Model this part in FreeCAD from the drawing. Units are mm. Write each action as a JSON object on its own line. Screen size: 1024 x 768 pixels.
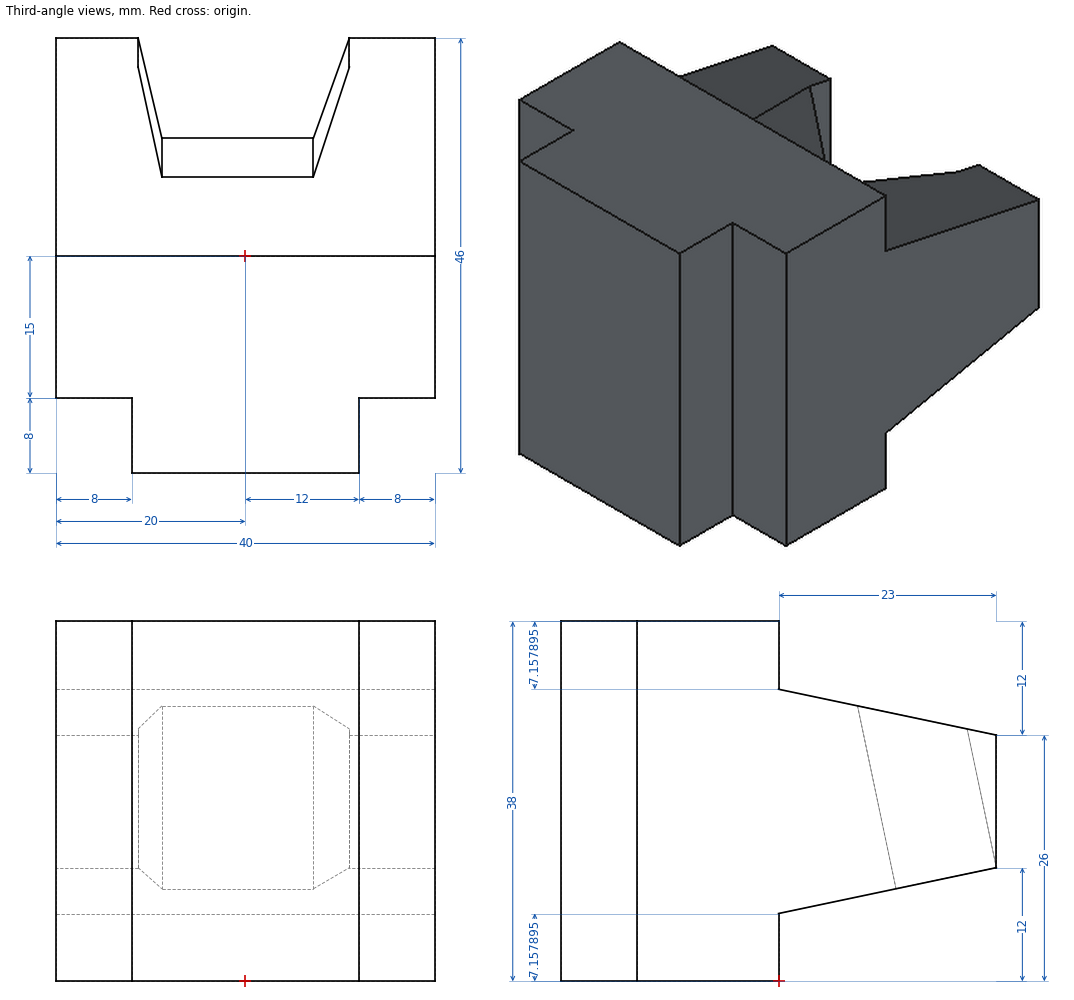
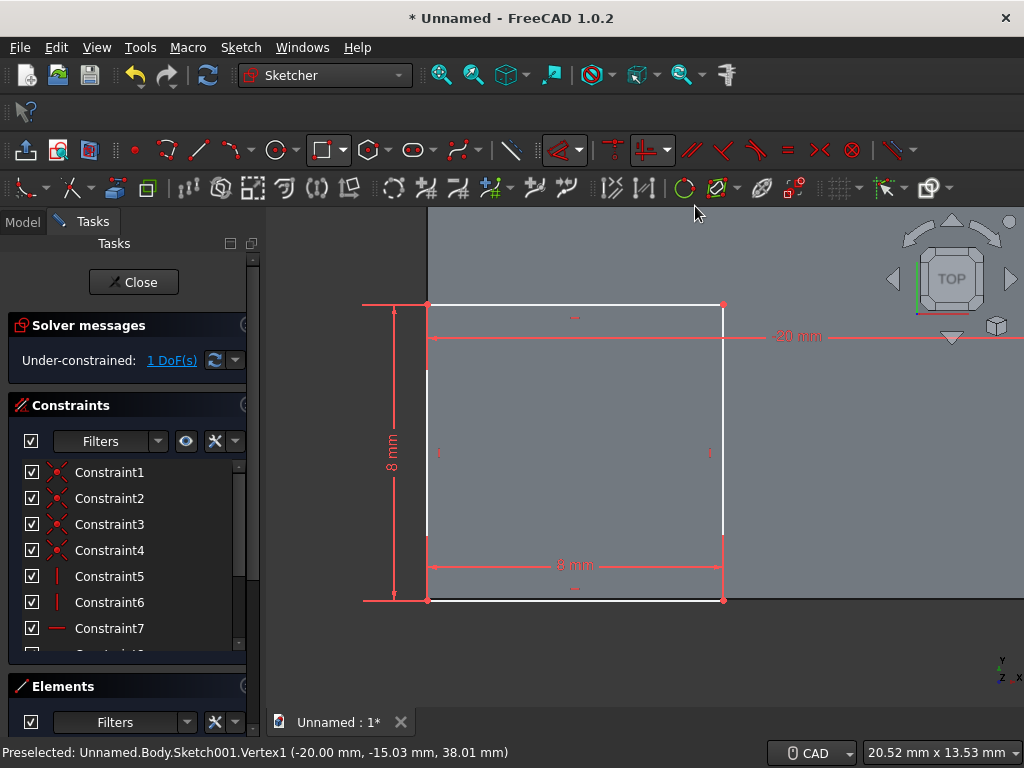
{"action": "left_click", "coordinate": [427, 305]}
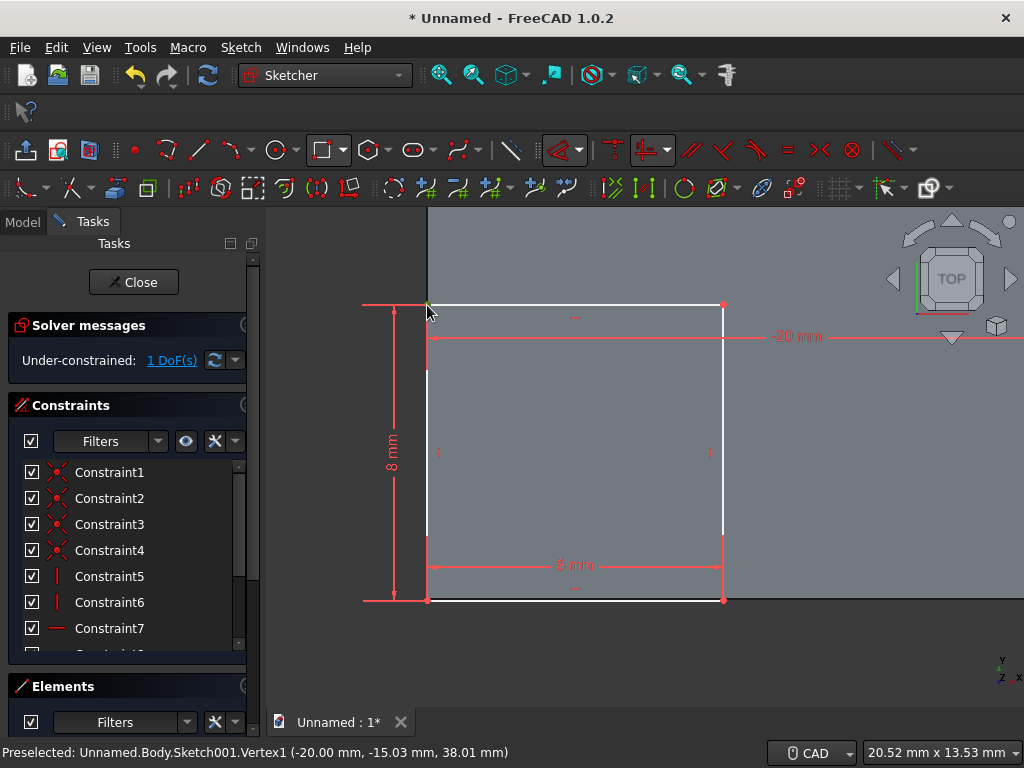
{"action": "left_click", "coordinate": [582, 150]}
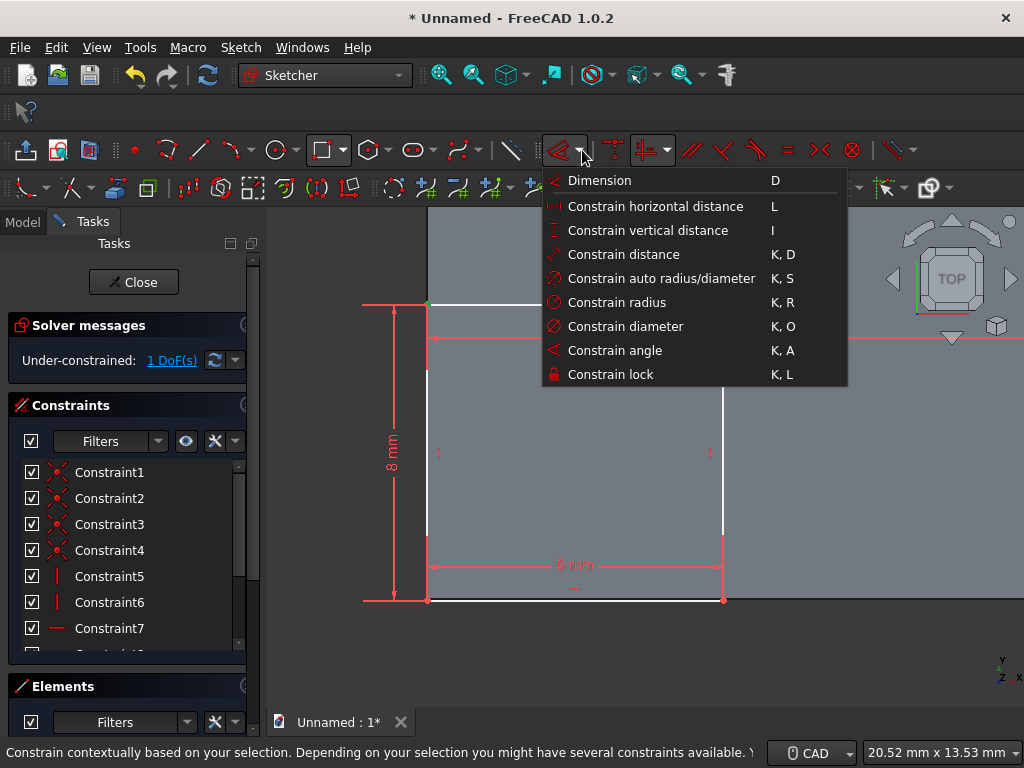
{"action": "left_click", "coordinate": [695, 230]}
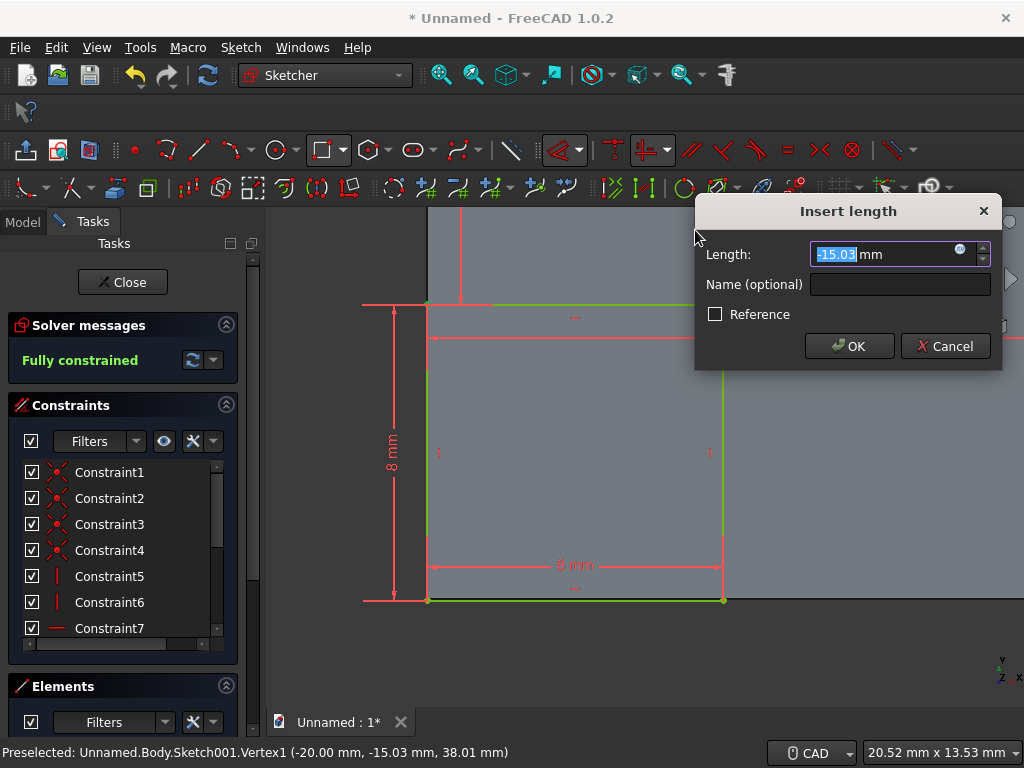
{"action": "type", "text": "-15"}
{"action": "key", "text": "Return"}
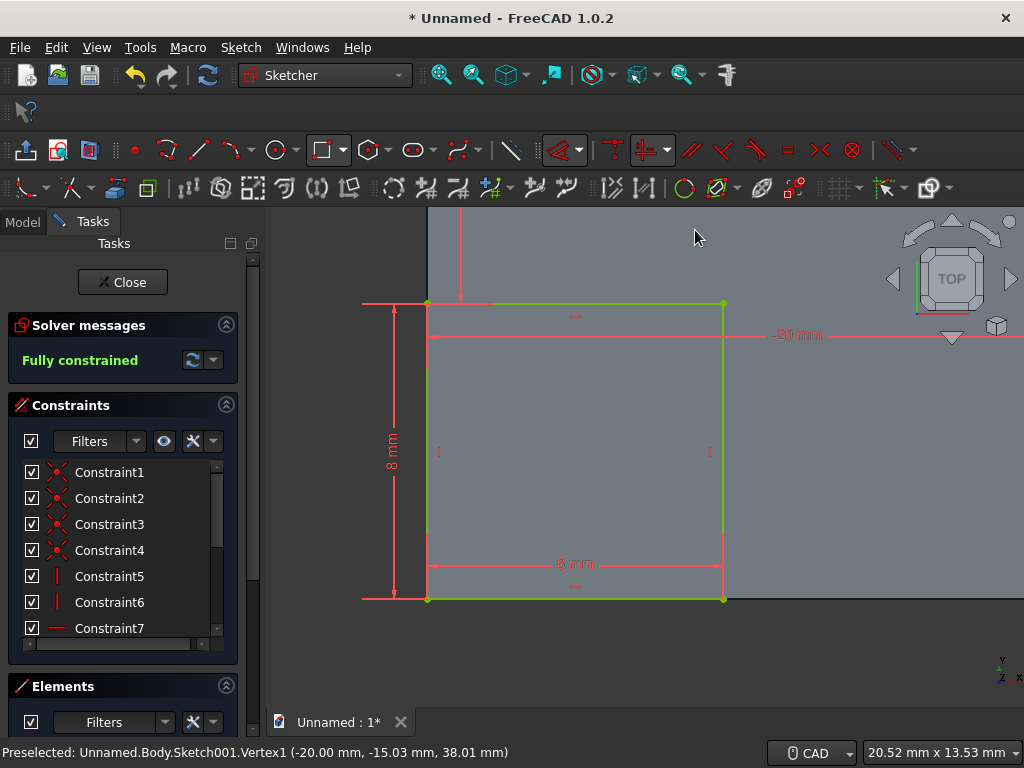
{"action": "left_click", "coordinate": [123, 282]}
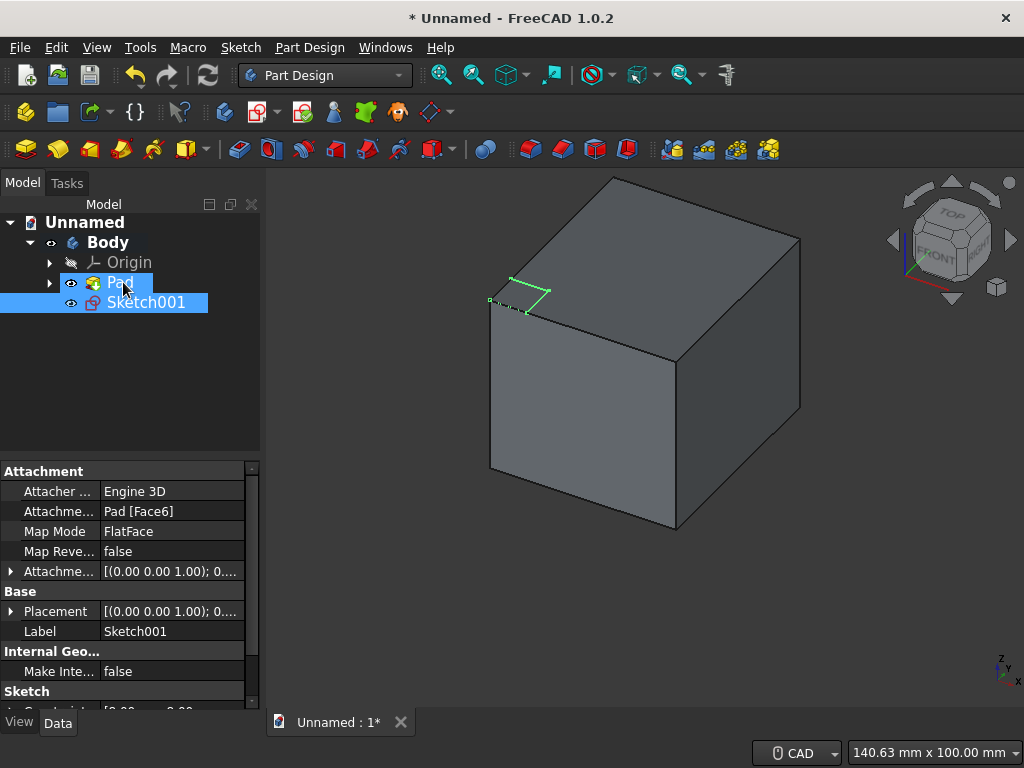
{"action": "left_click", "coordinate": [240, 150]}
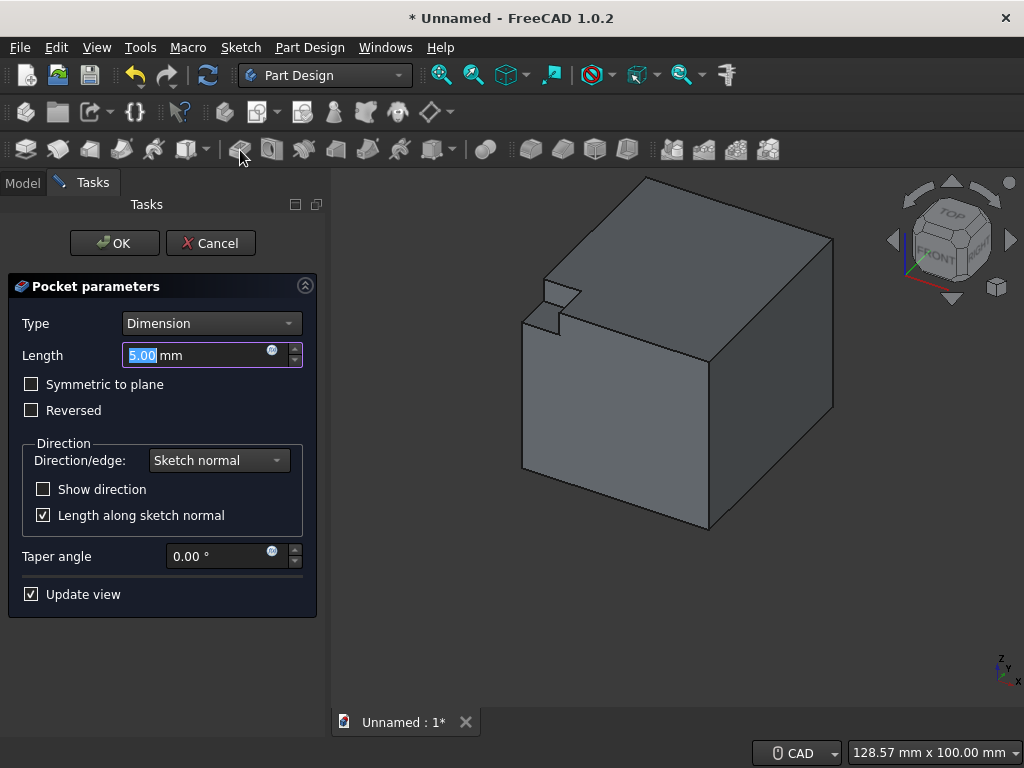
{"action": "left_click", "coordinate": [212, 324]}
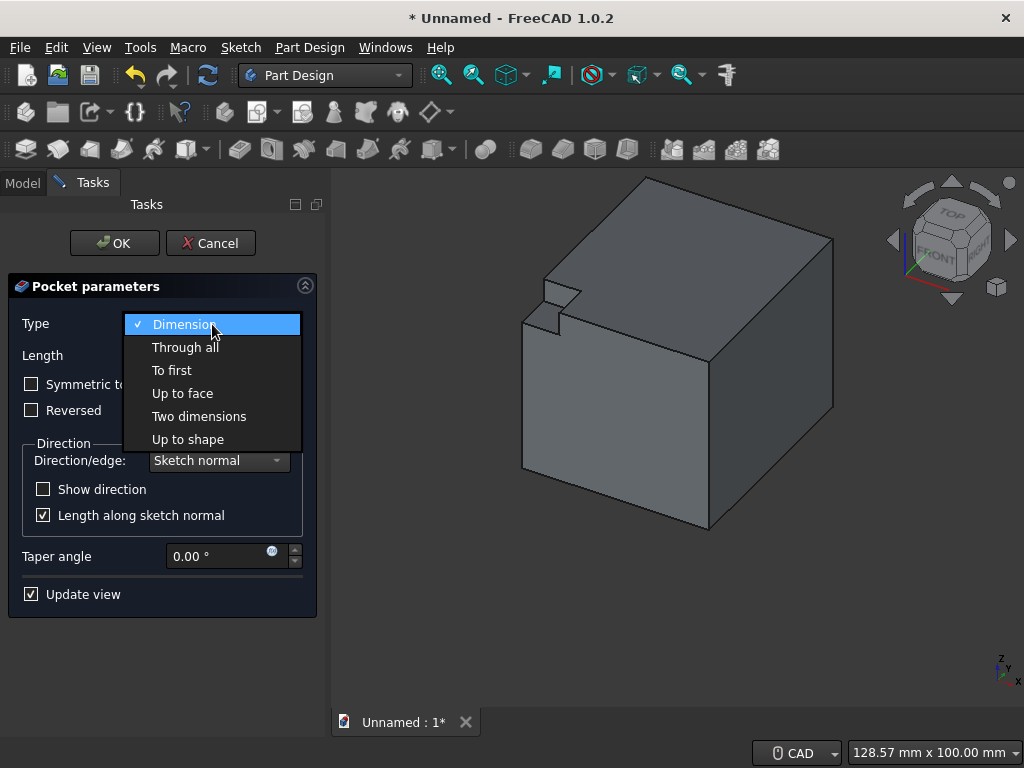
{"action": "left_click", "coordinate": [212, 348]}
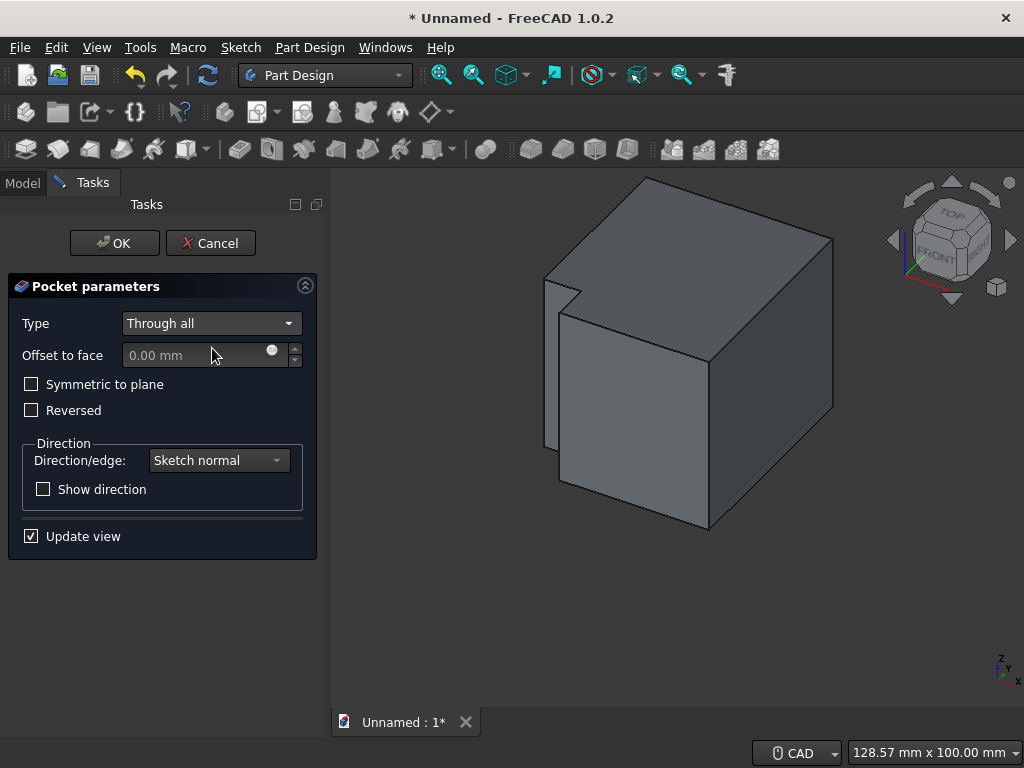
{"action": "left_click", "coordinate": [115, 243]}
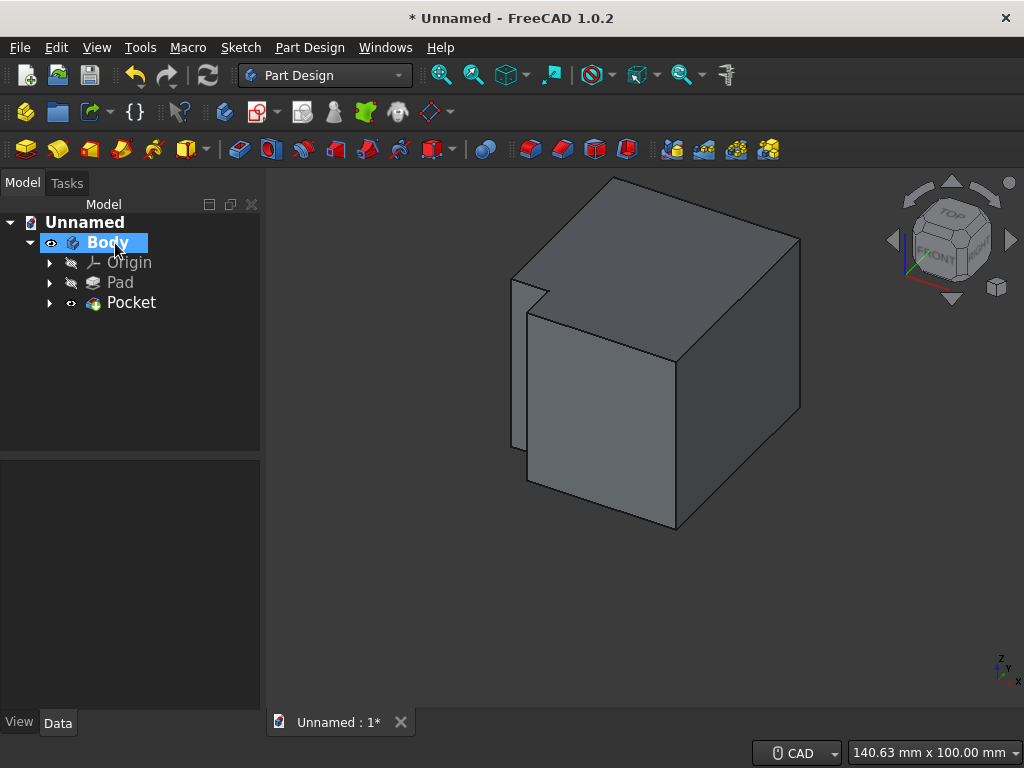
{"action": "left_click", "coordinate": [645, 269]}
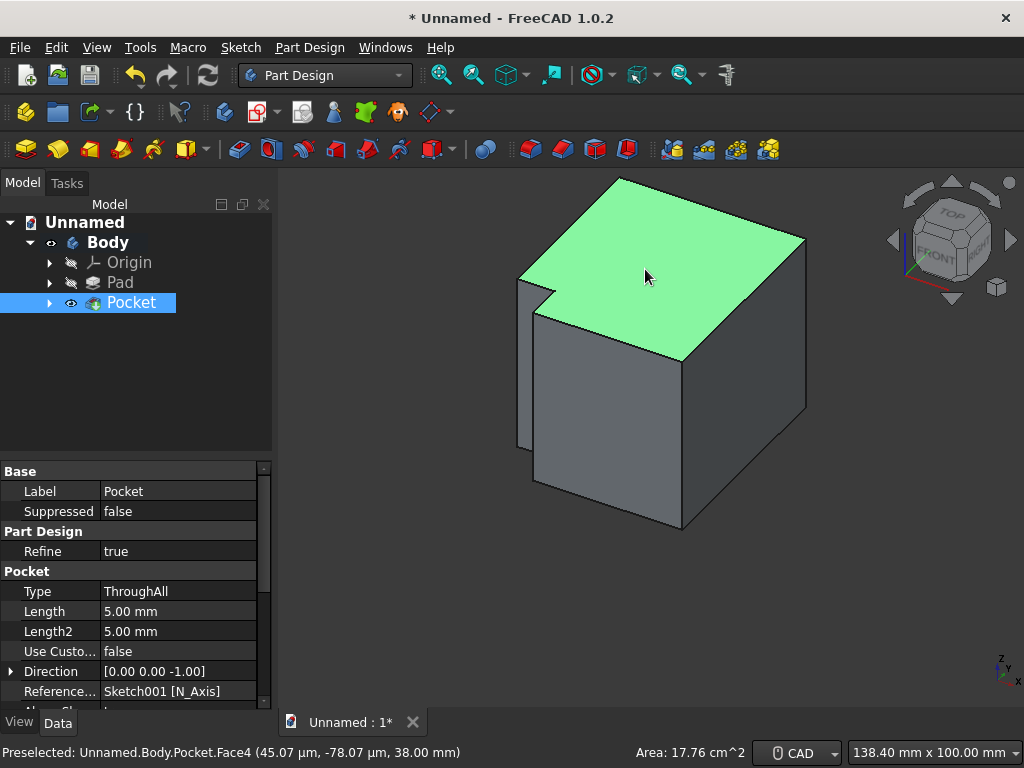
{"action": "left_click", "coordinate": [258, 112]}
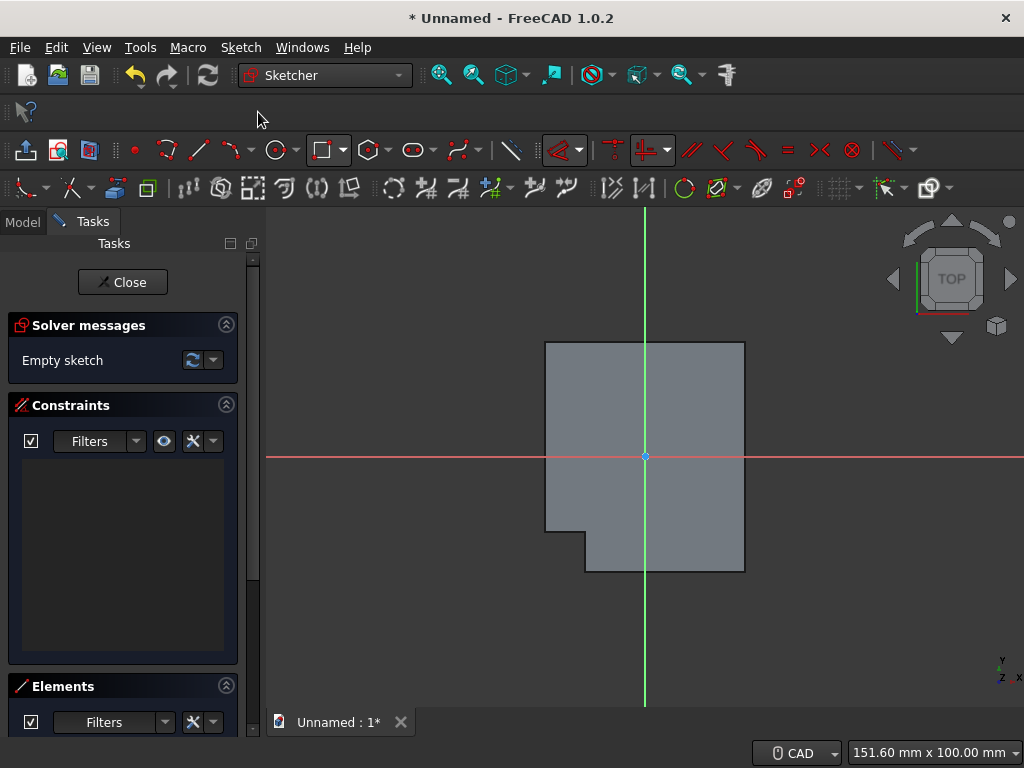
{"action": "scroll", "coordinate": [748, 567], "scroll_direction": "up", "scroll_amount": 10}